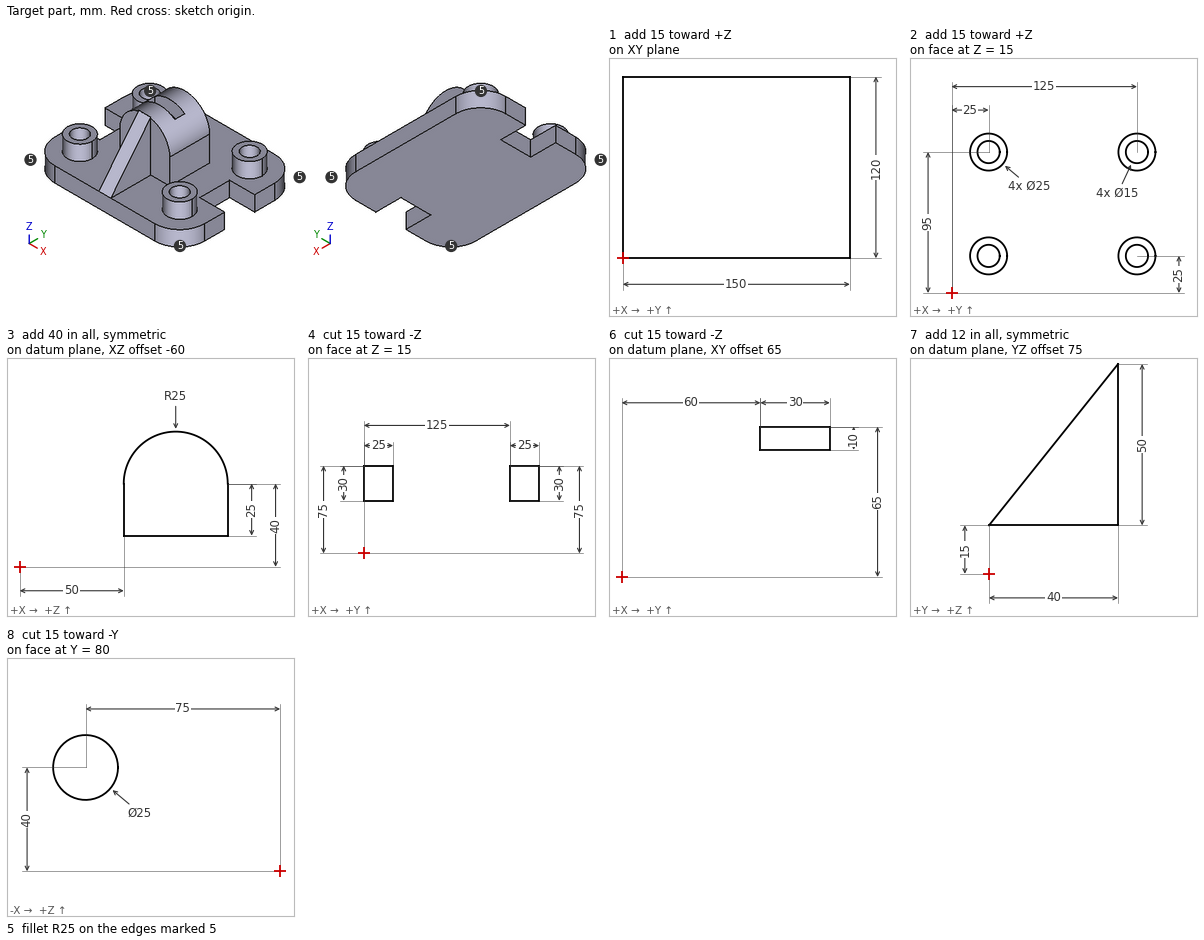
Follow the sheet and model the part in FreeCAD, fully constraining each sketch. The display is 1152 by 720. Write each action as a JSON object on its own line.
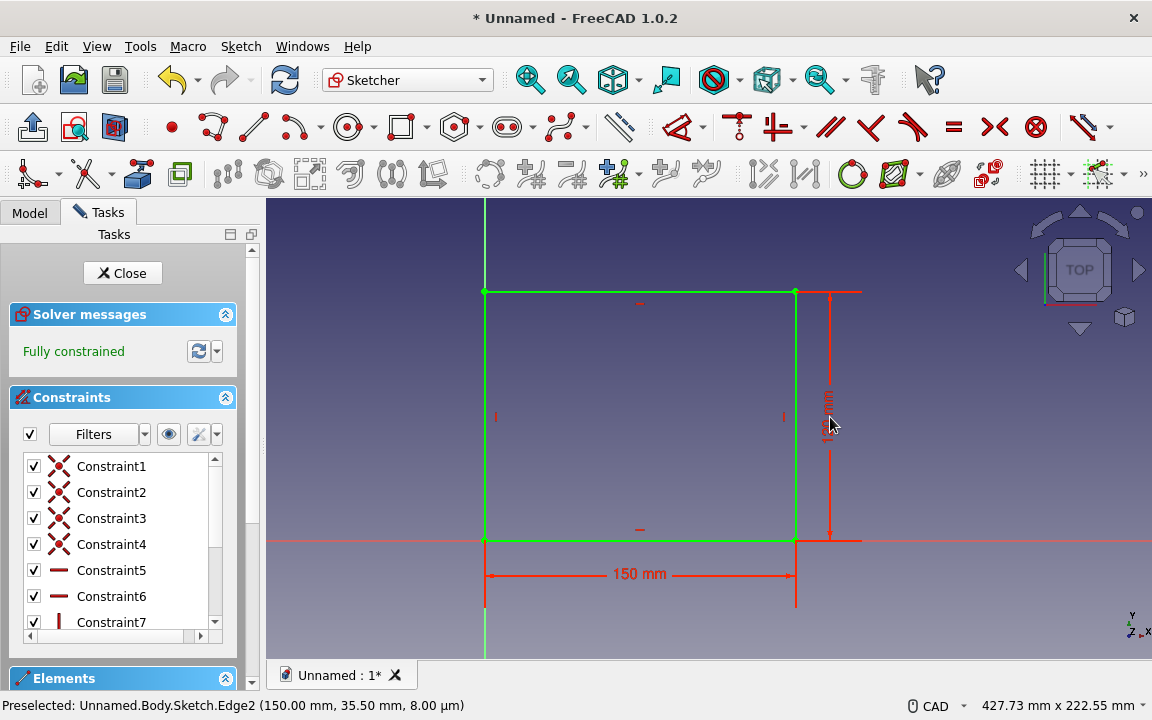
{"action": "left_click", "coordinate": [123, 273]}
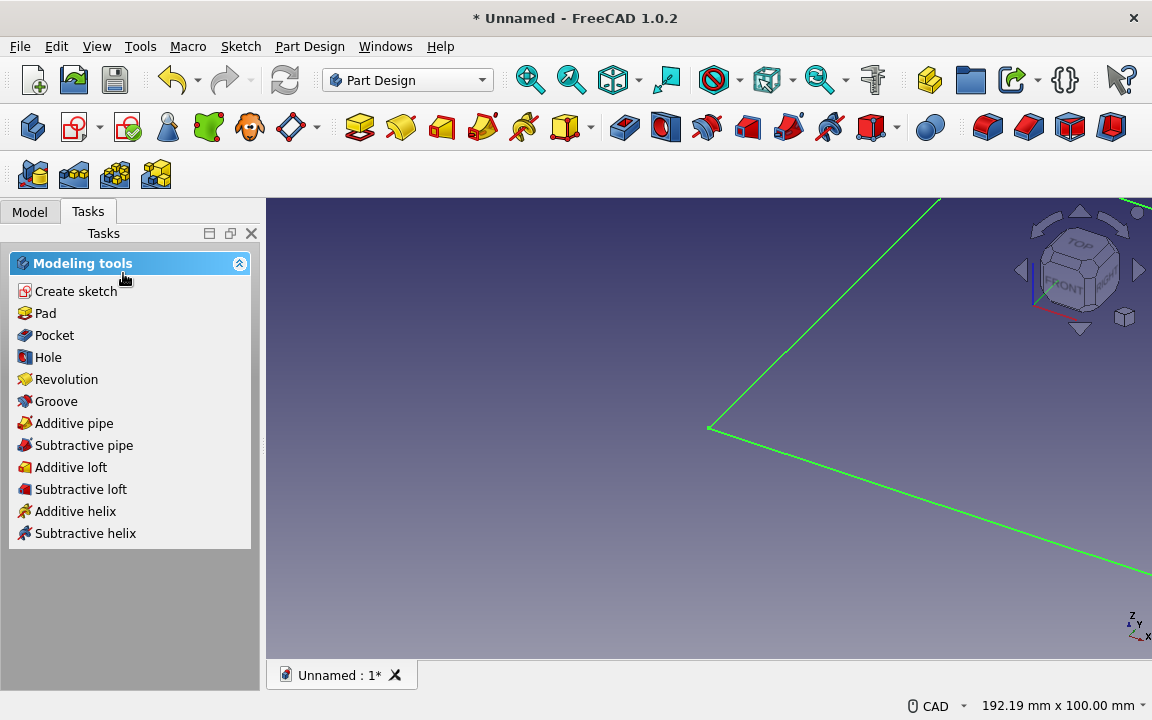
{"action": "left_click", "coordinate": [360, 128]}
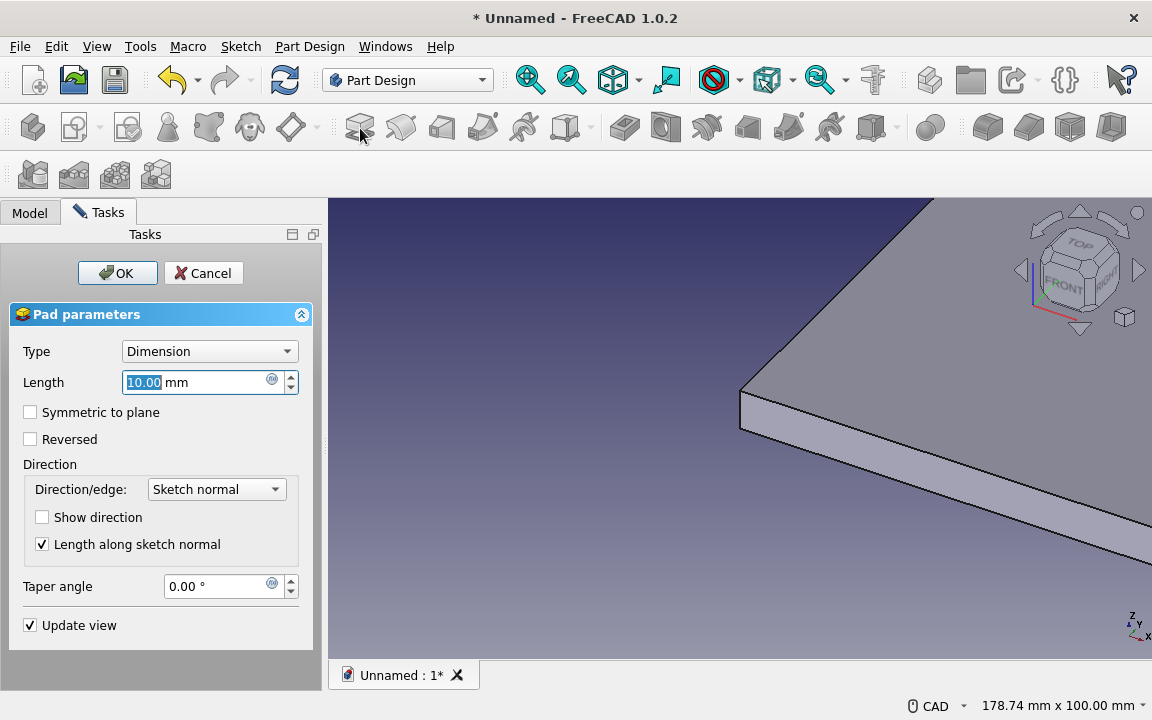
{"action": "type", "text": "15"}
{"action": "key", "text": "Tab"}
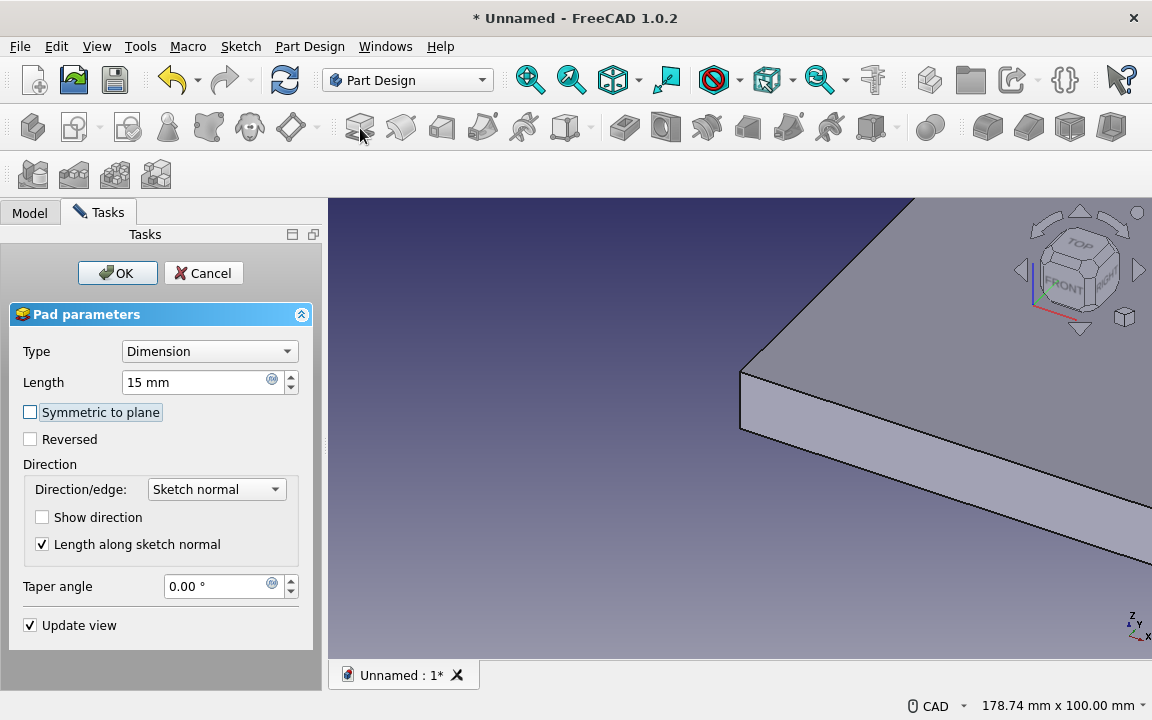
{"action": "left_click", "coordinate": [118, 273]}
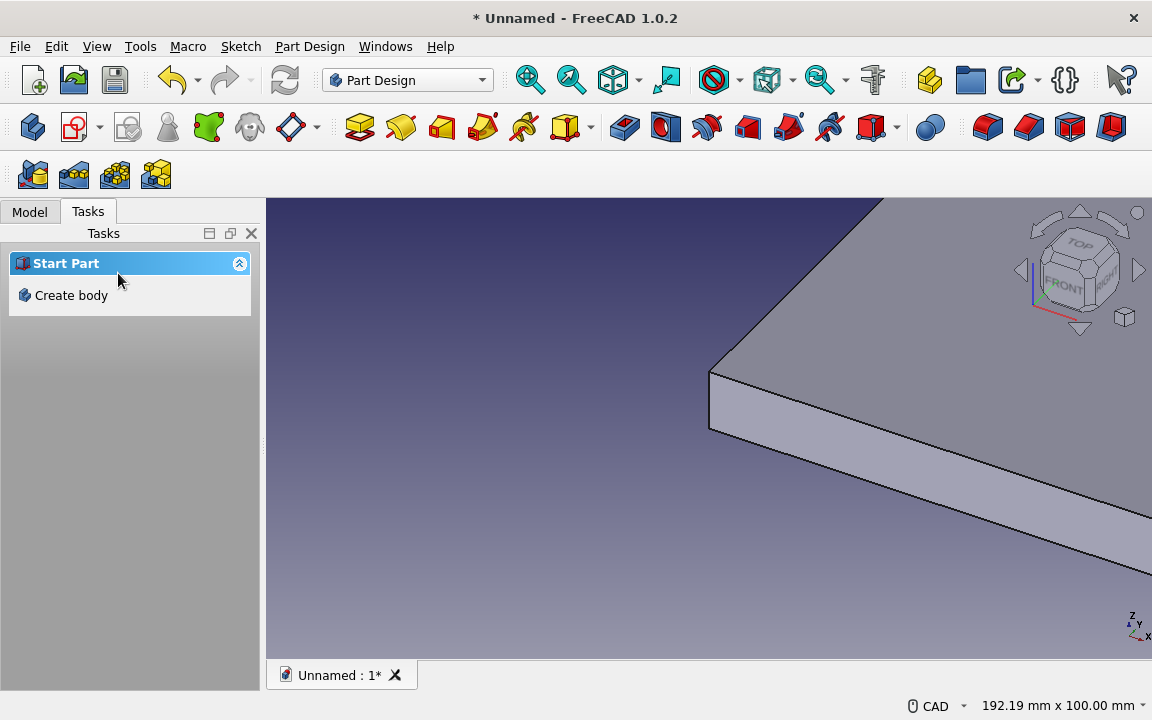
{"action": "left_click", "coordinate": [531, 80]}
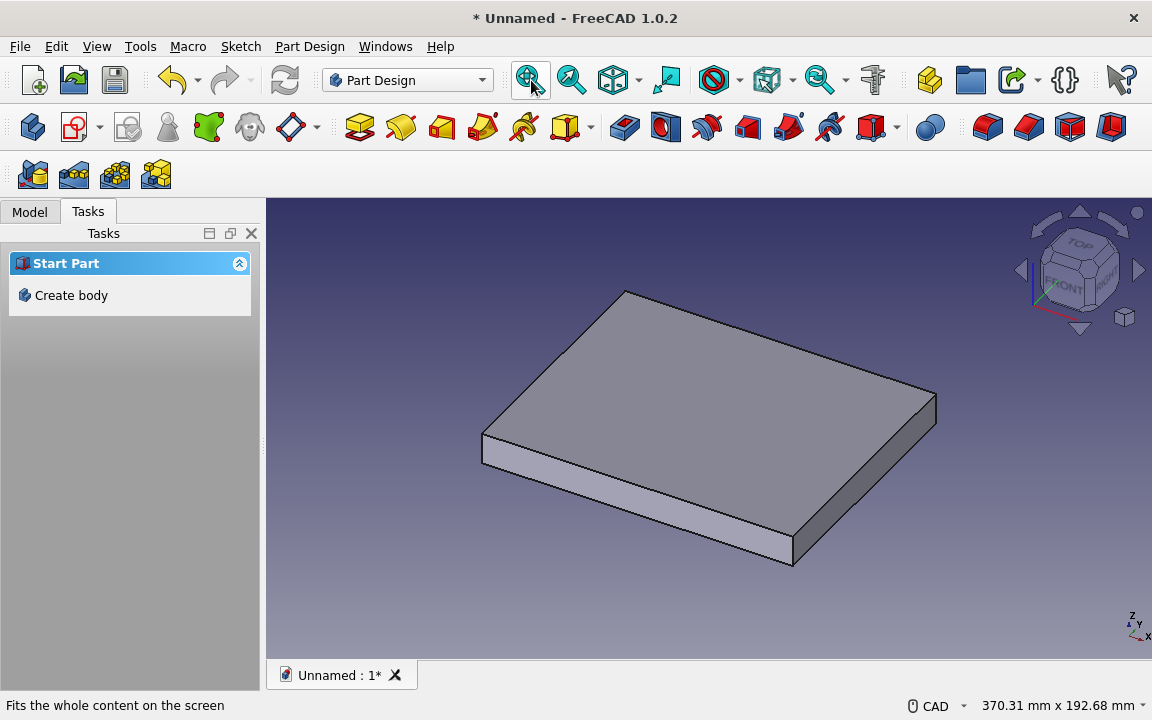
{"action": "left_click", "coordinate": [709, 413]}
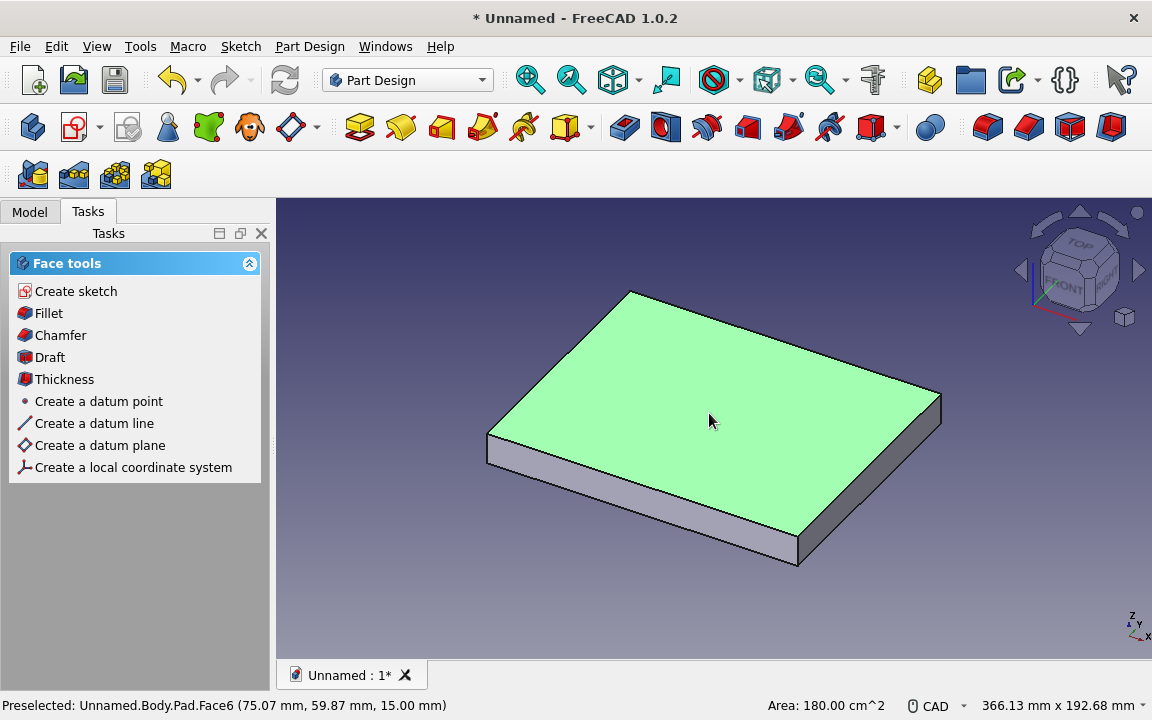
{"action": "left_click", "coordinate": [74, 128]}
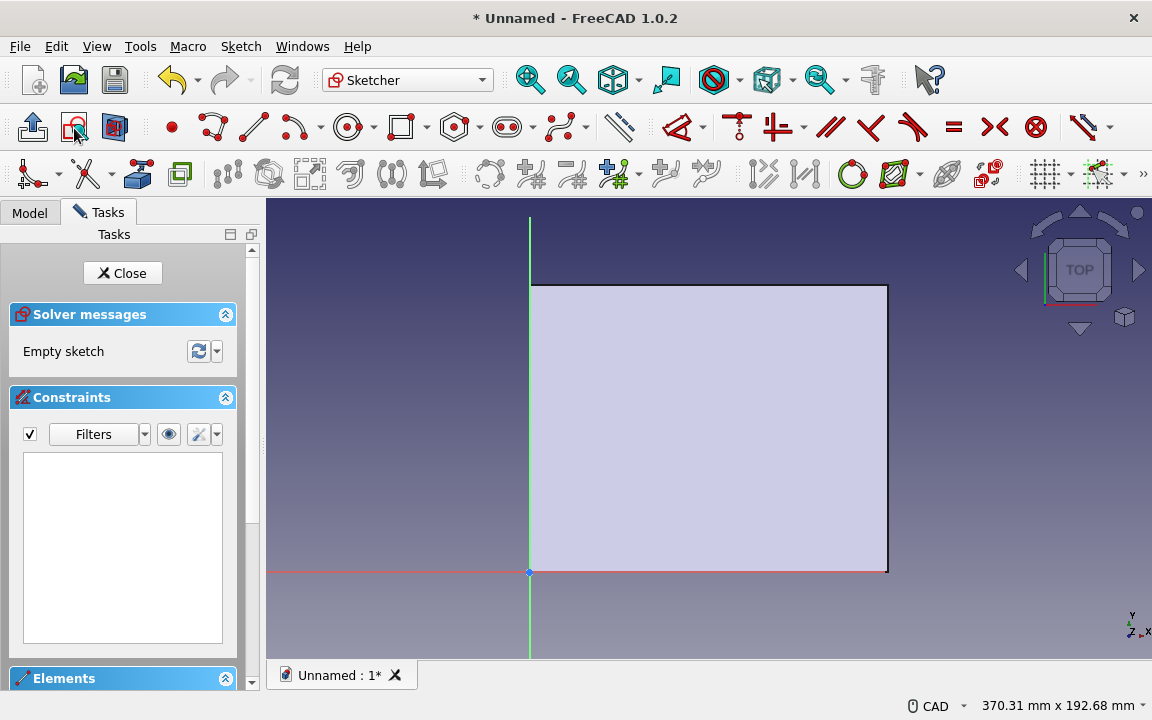
{"action": "left_click", "coordinate": [348, 128]}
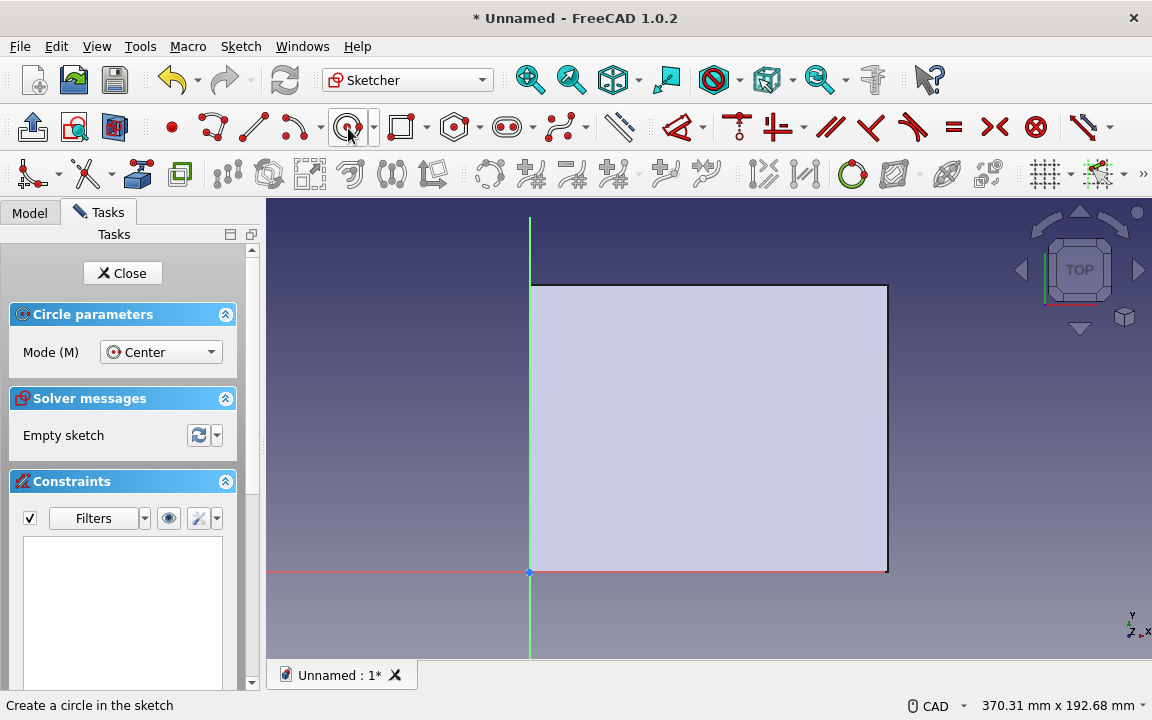
{"action": "left_click", "coordinate": [589, 345]}
{"action": "left_click", "coordinate": [611, 324]}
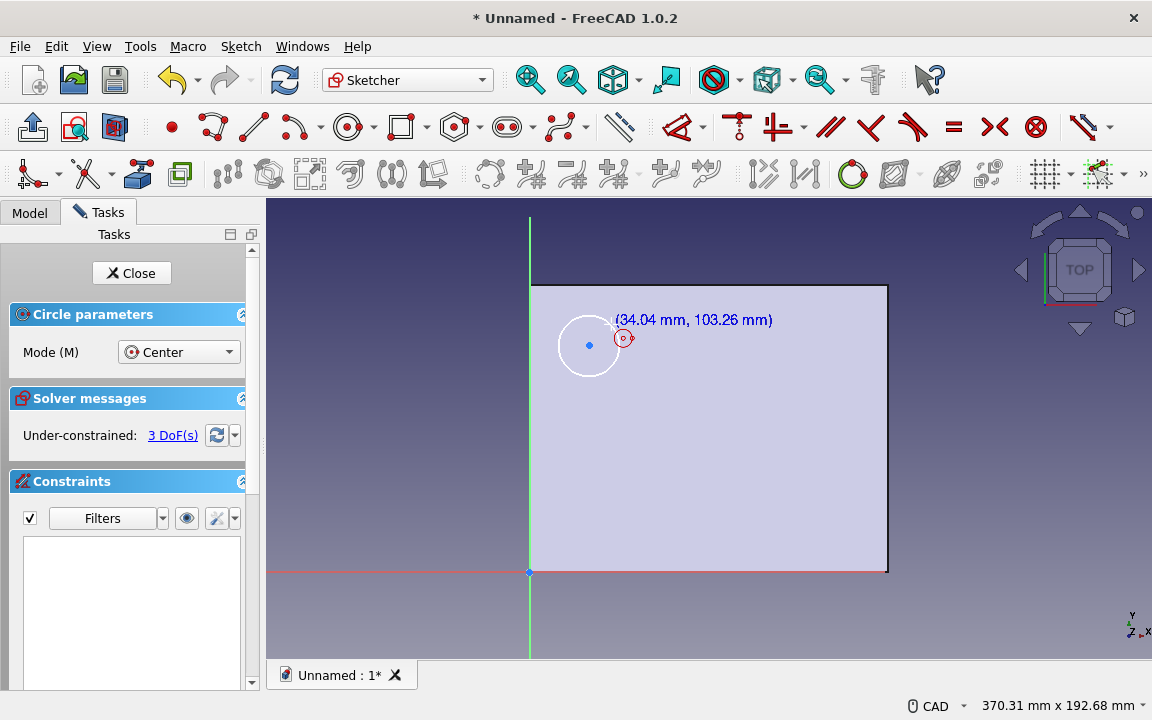
{"action": "left_click", "coordinate": [829, 345]}
{"action": "left_click", "coordinate": [850, 324]}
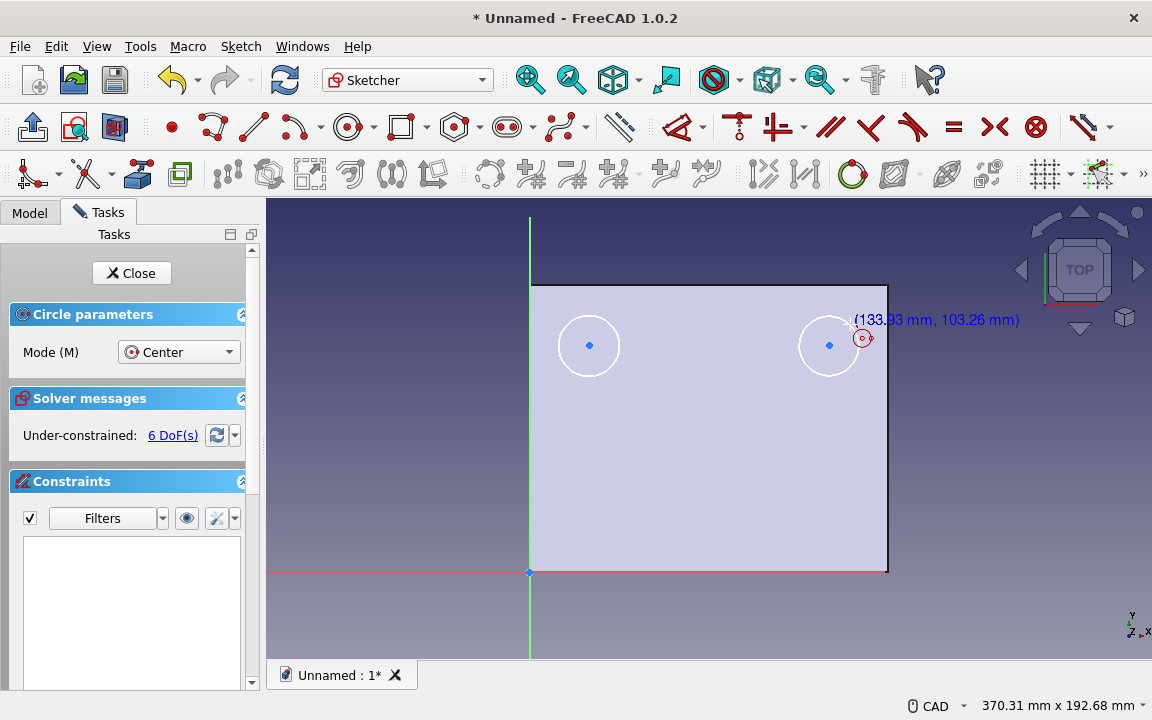
{"action": "left_click", "coordinate": [829, 512]}
{"action": "left_click", "coordinate": [850, 491]}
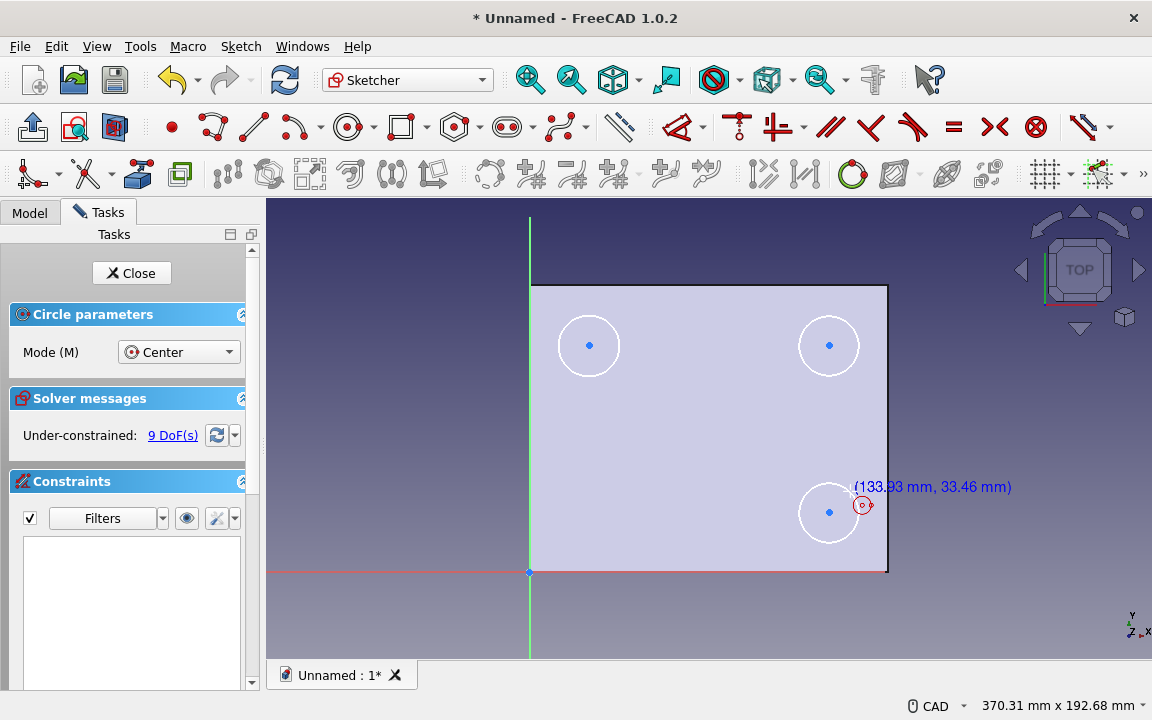
{"action": "left_click", "coordinate": [589, 512]}
{"action": "left_click", "coordinate": [611, 491]}